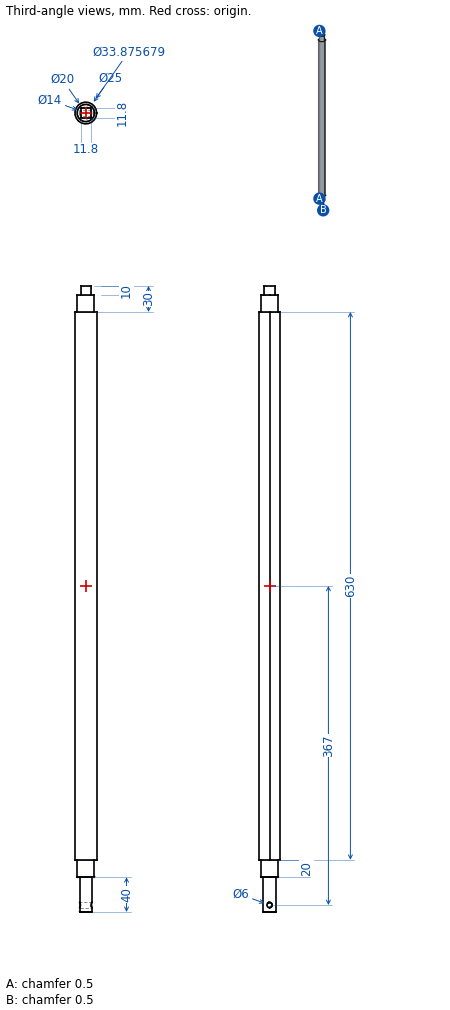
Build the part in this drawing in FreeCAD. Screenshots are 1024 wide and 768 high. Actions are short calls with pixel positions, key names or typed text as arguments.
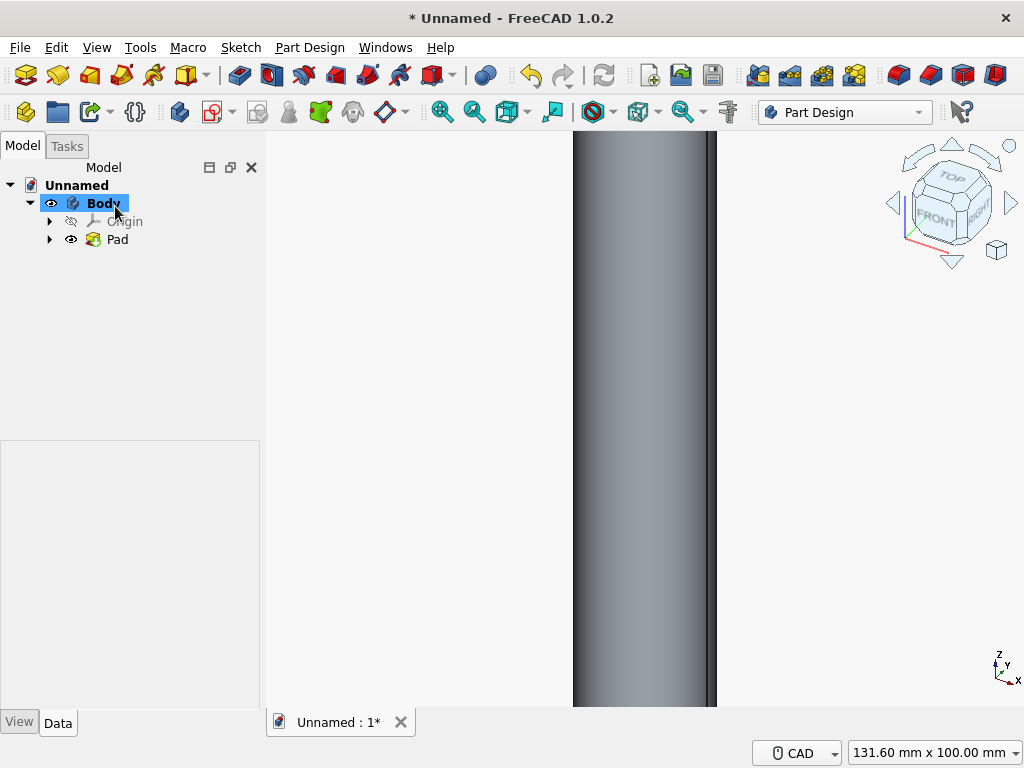
click(444, 112)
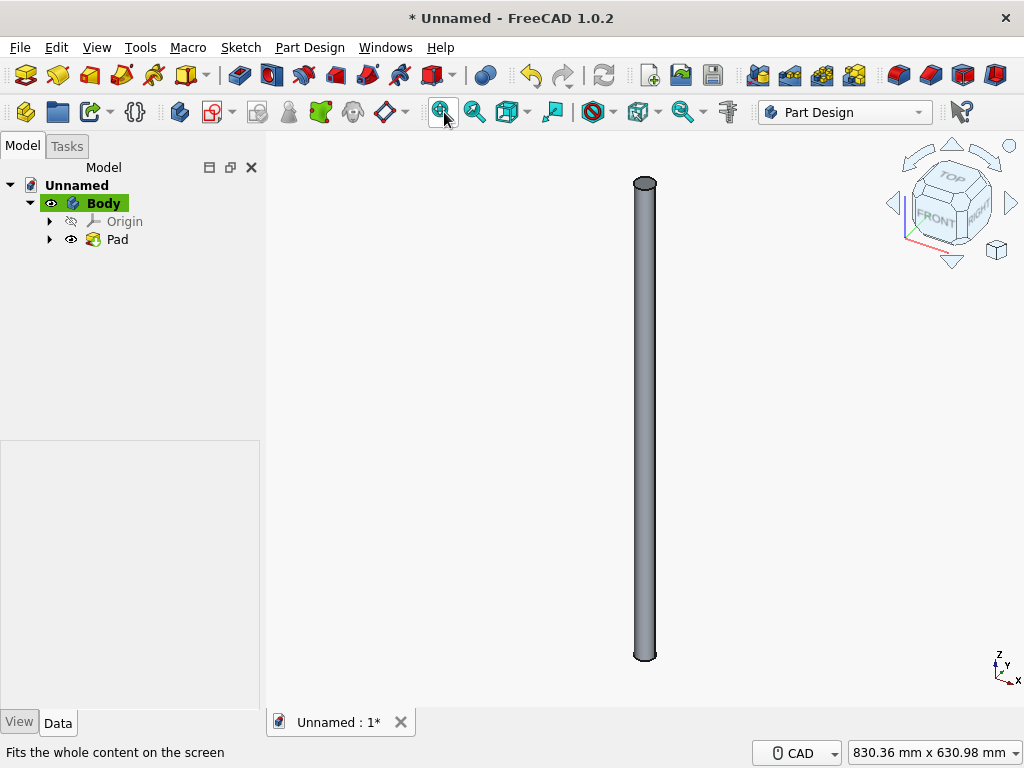
click(644, 180)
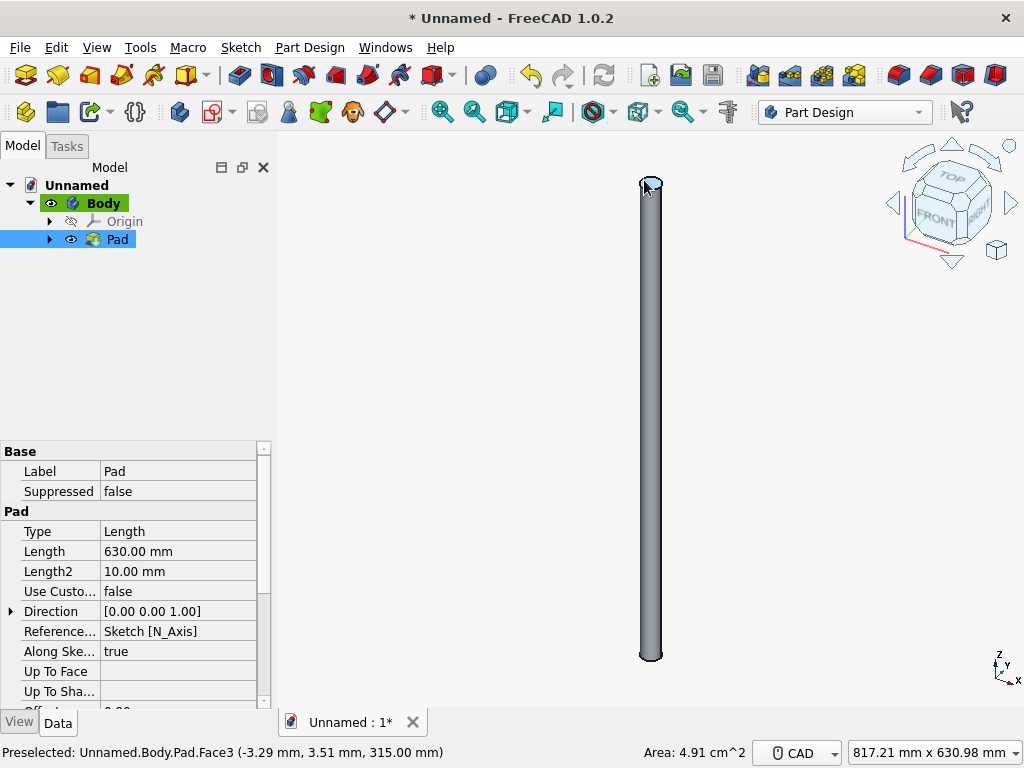
click(212, 112)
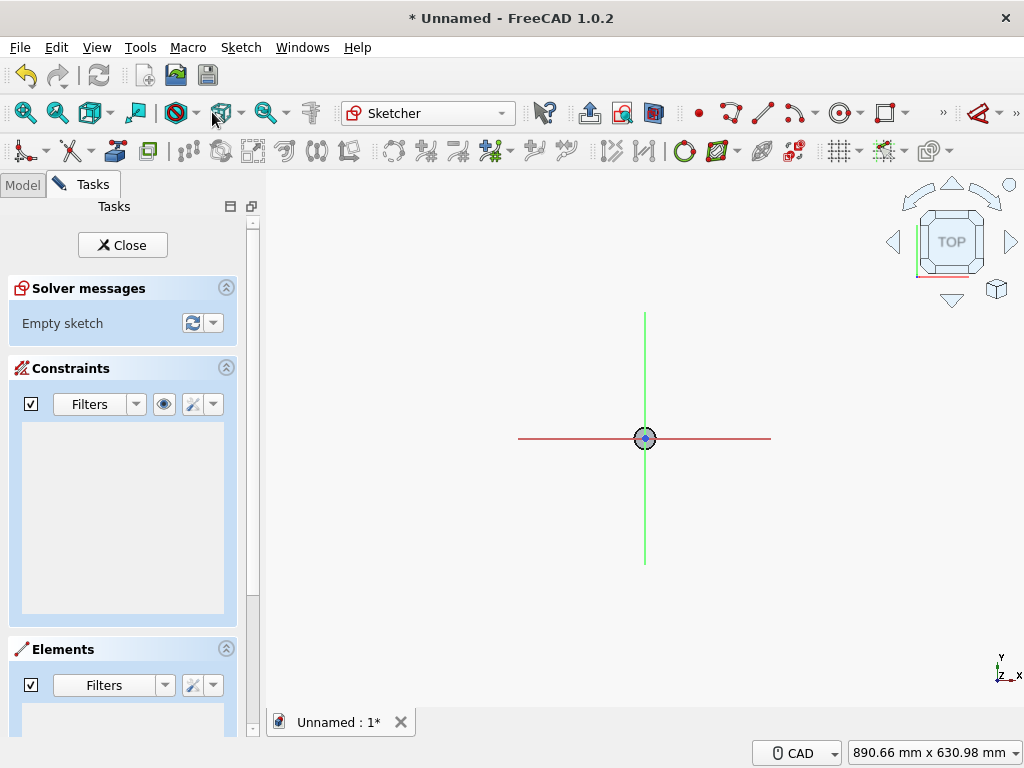
scroll(649, 438, up, 15)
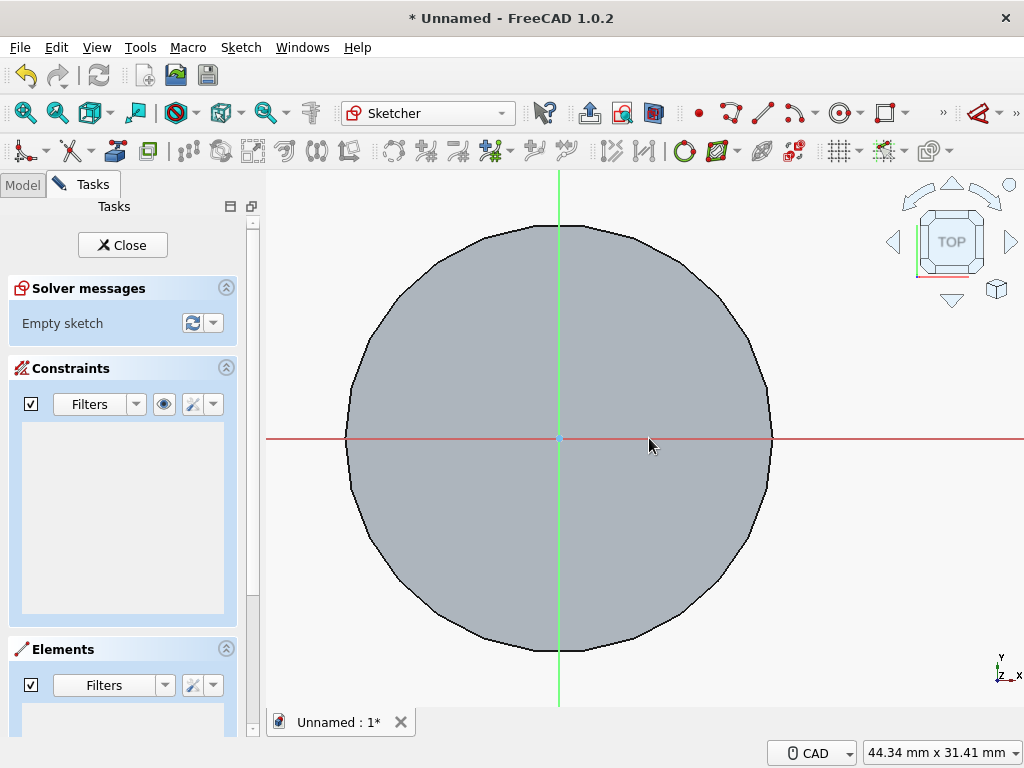
click(840, 114)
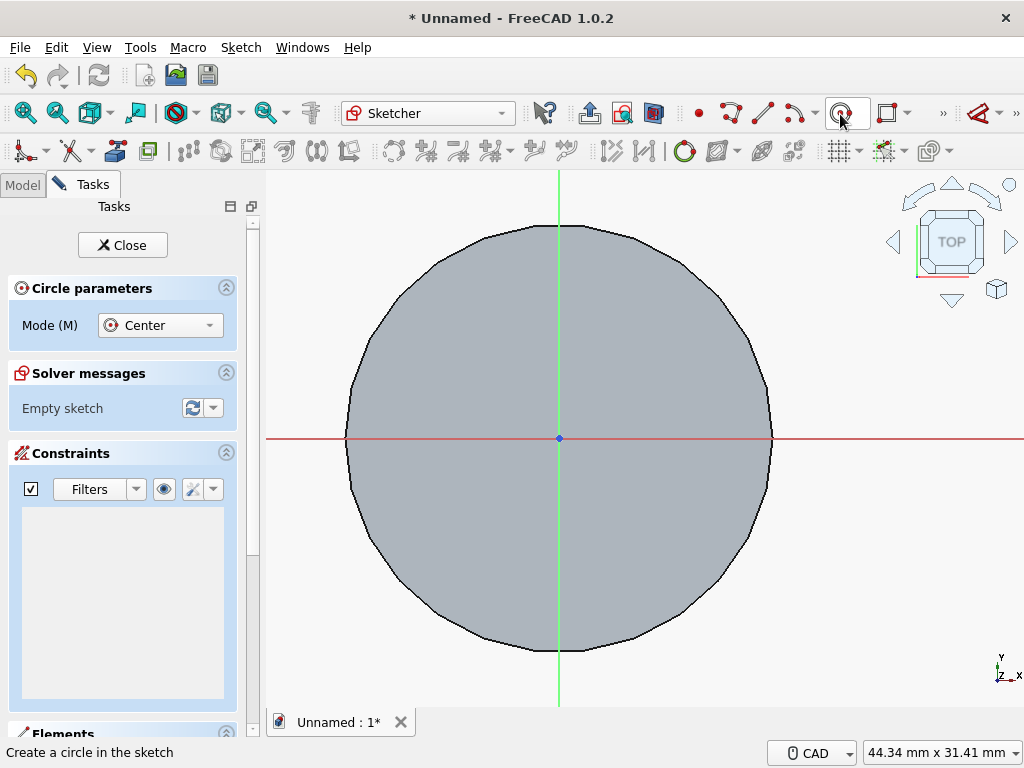
click(559, 438)
move(680, 318)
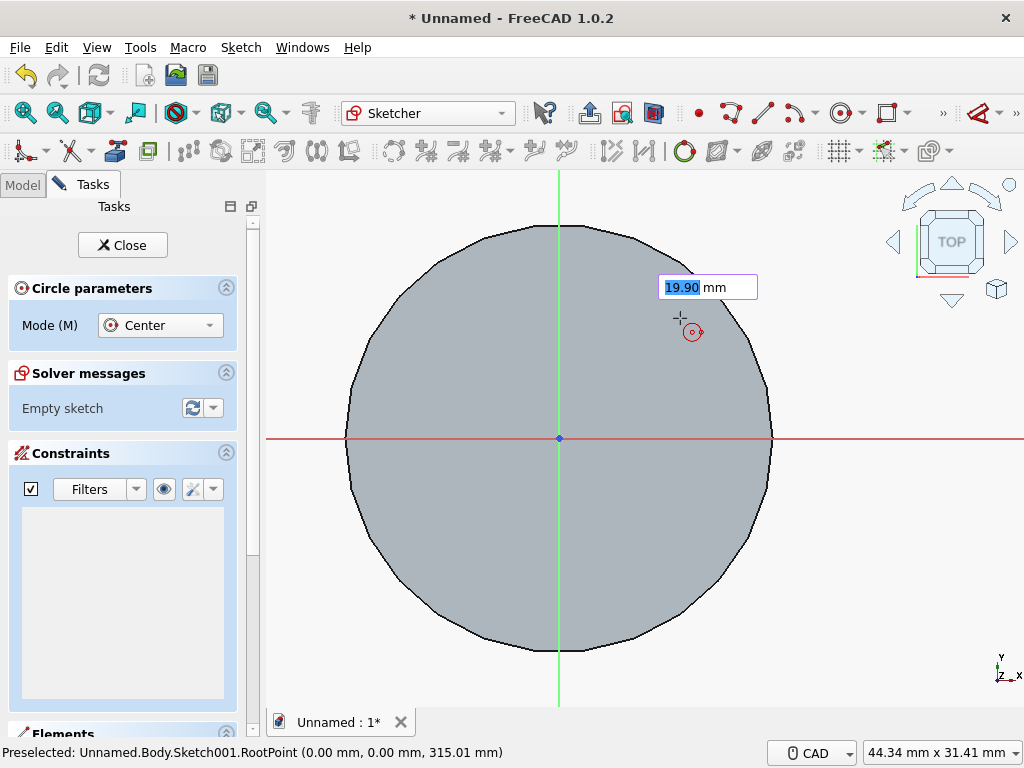
text(20)
key(Return)
key(Escape)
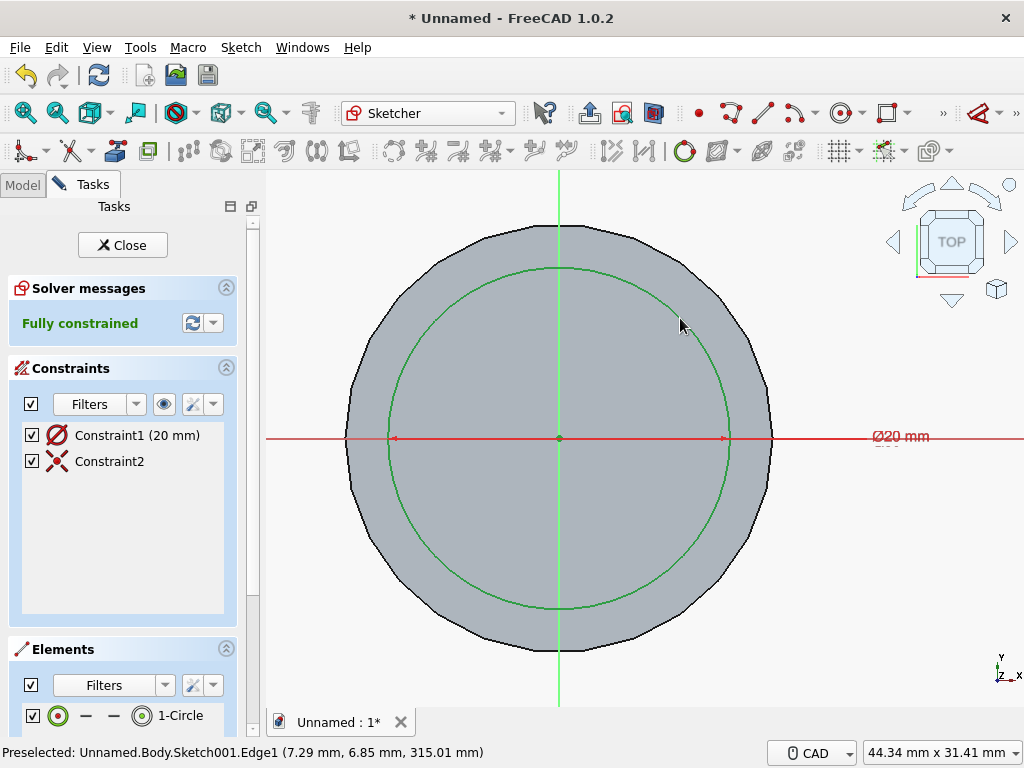
click(123, 245)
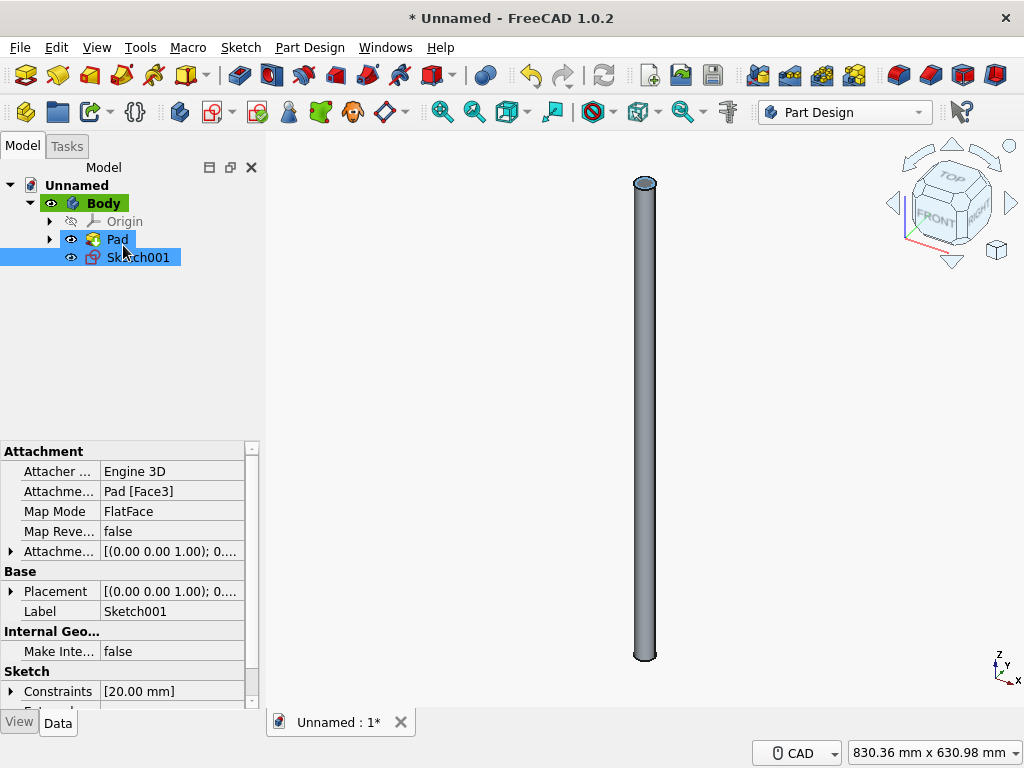
click(26, 76)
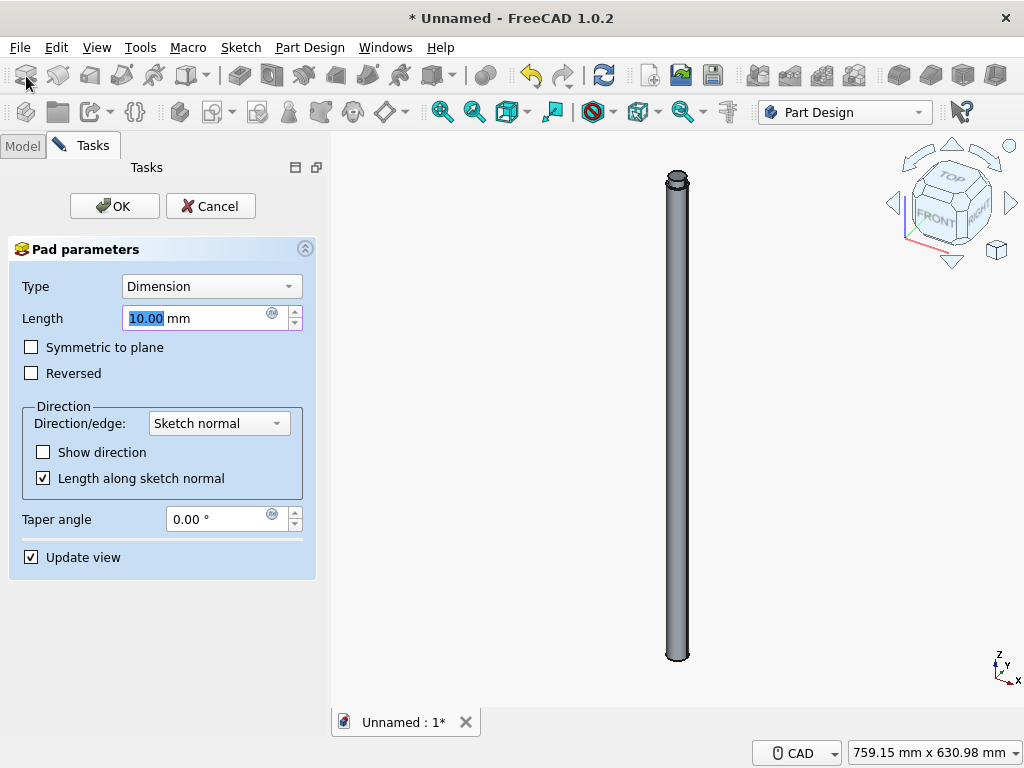
text(30)
key(Tab)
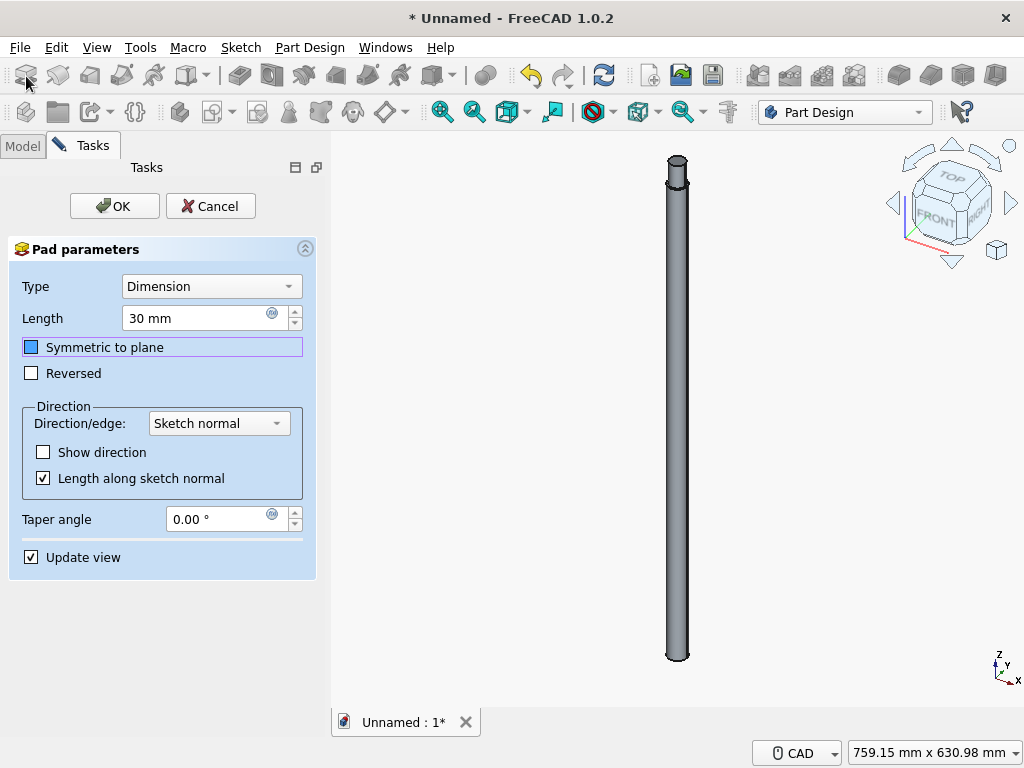
click(115, 206)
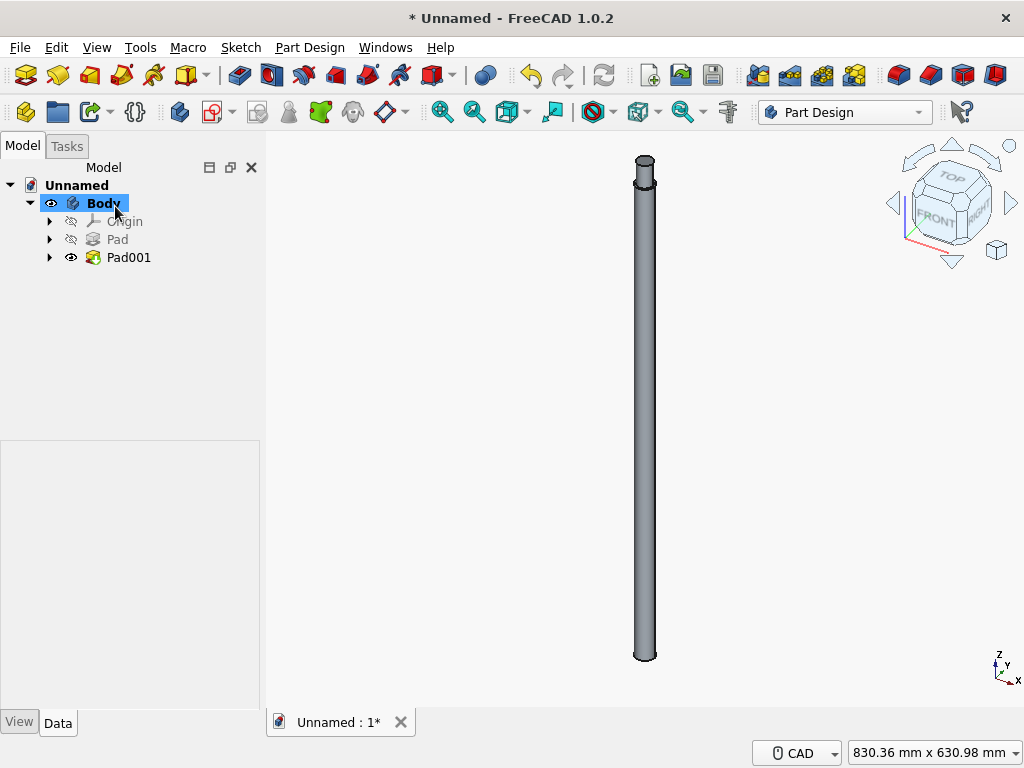
click(50, 221)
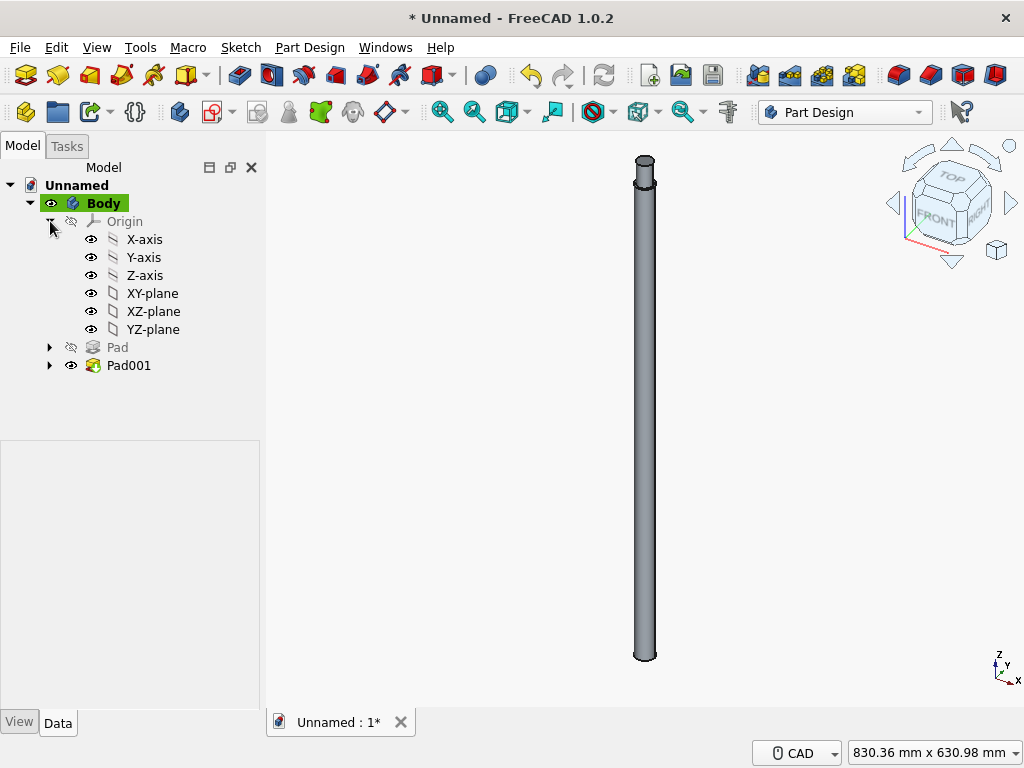
click(136, 293)